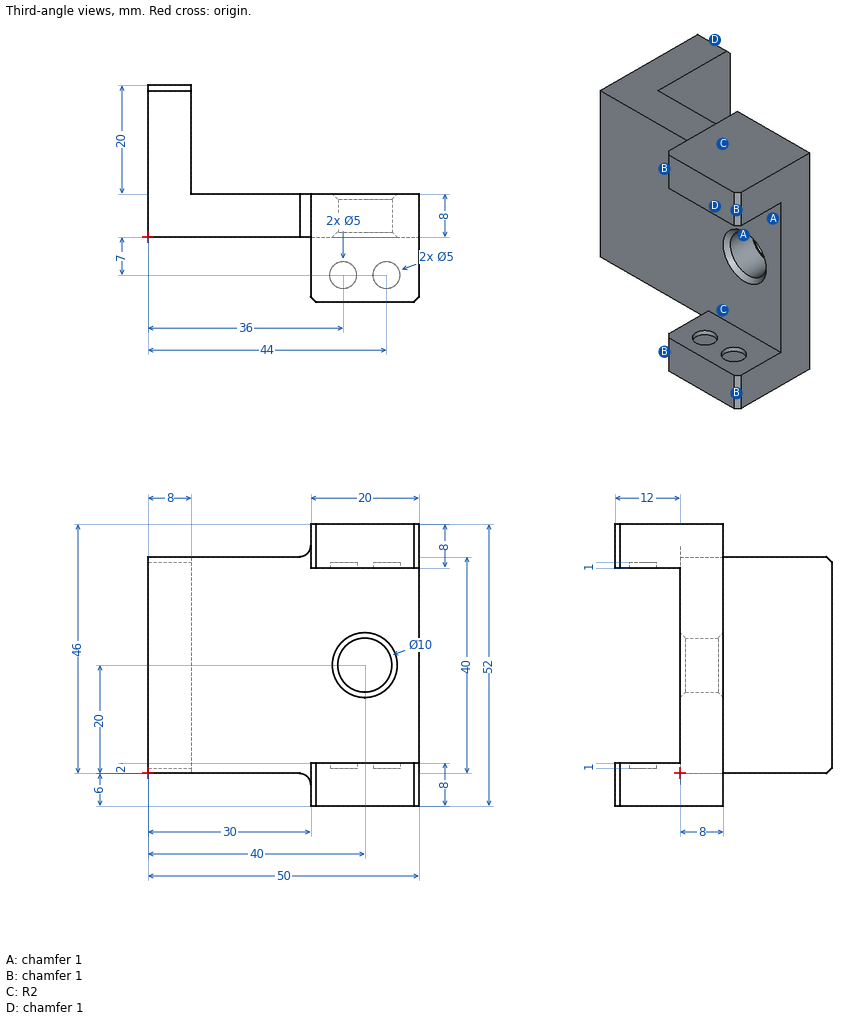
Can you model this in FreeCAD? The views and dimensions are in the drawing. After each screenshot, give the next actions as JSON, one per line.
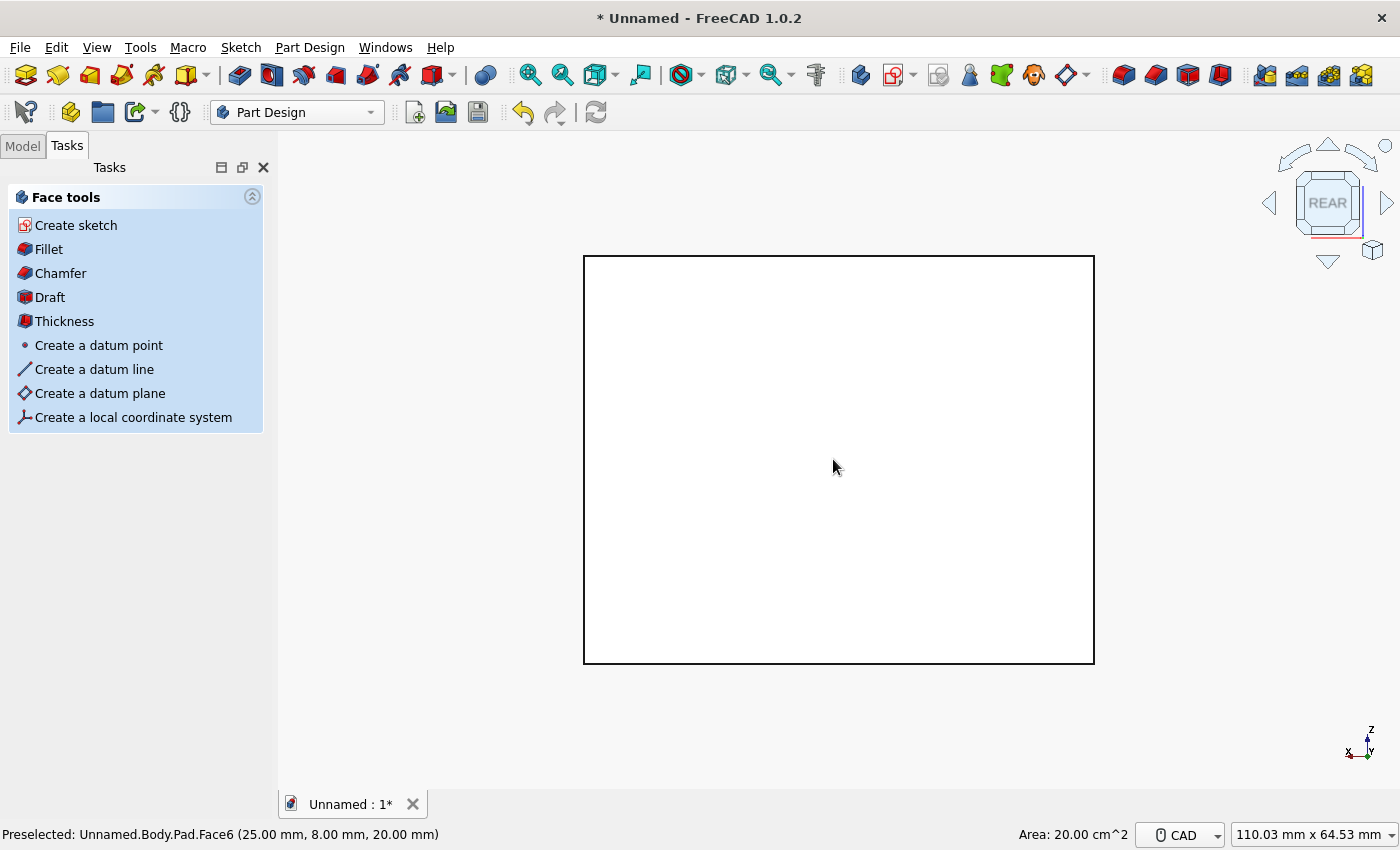
{"action": "left_click", "coordinate": [894, 76]}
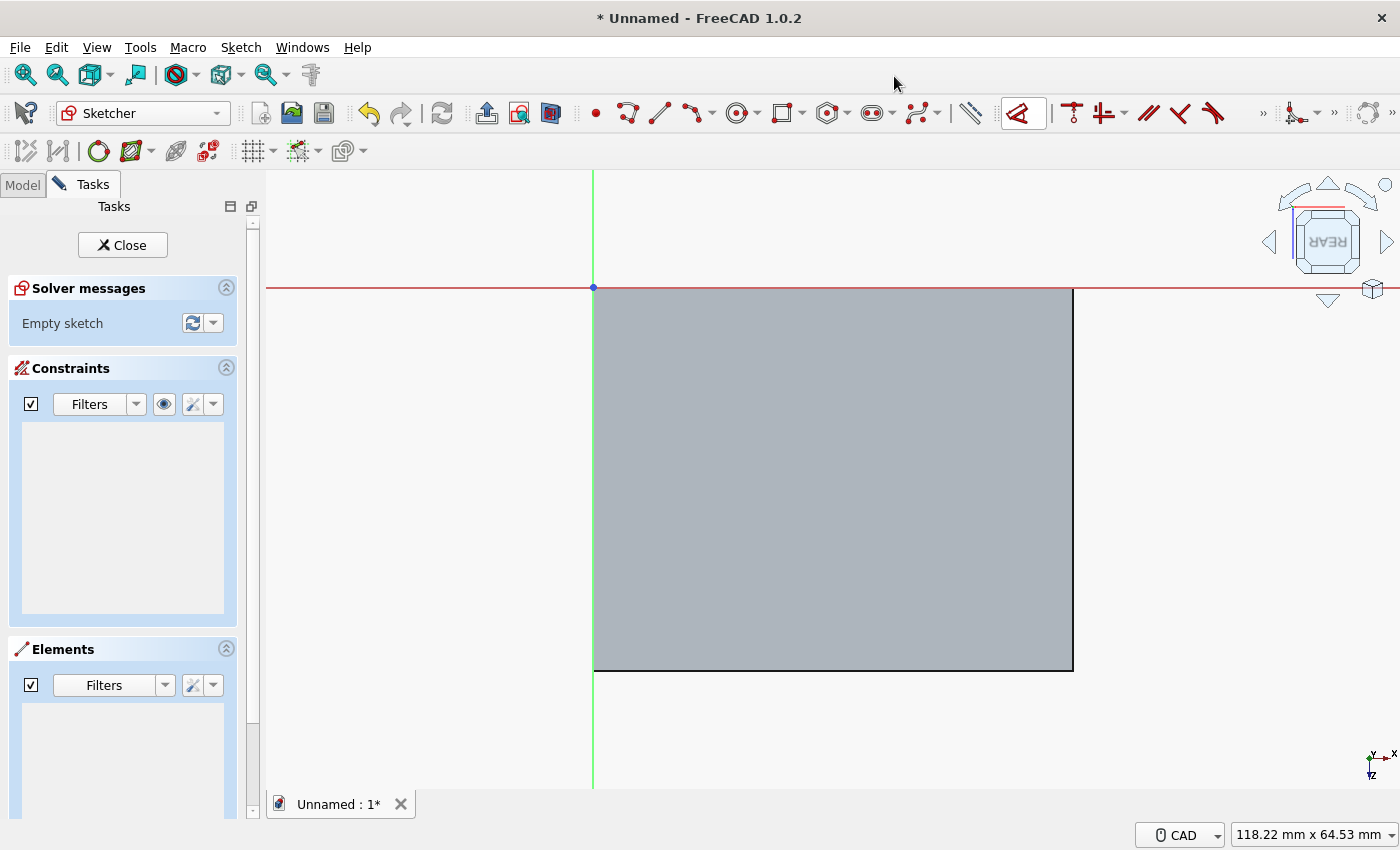
{"action": "key", "text": "g r"}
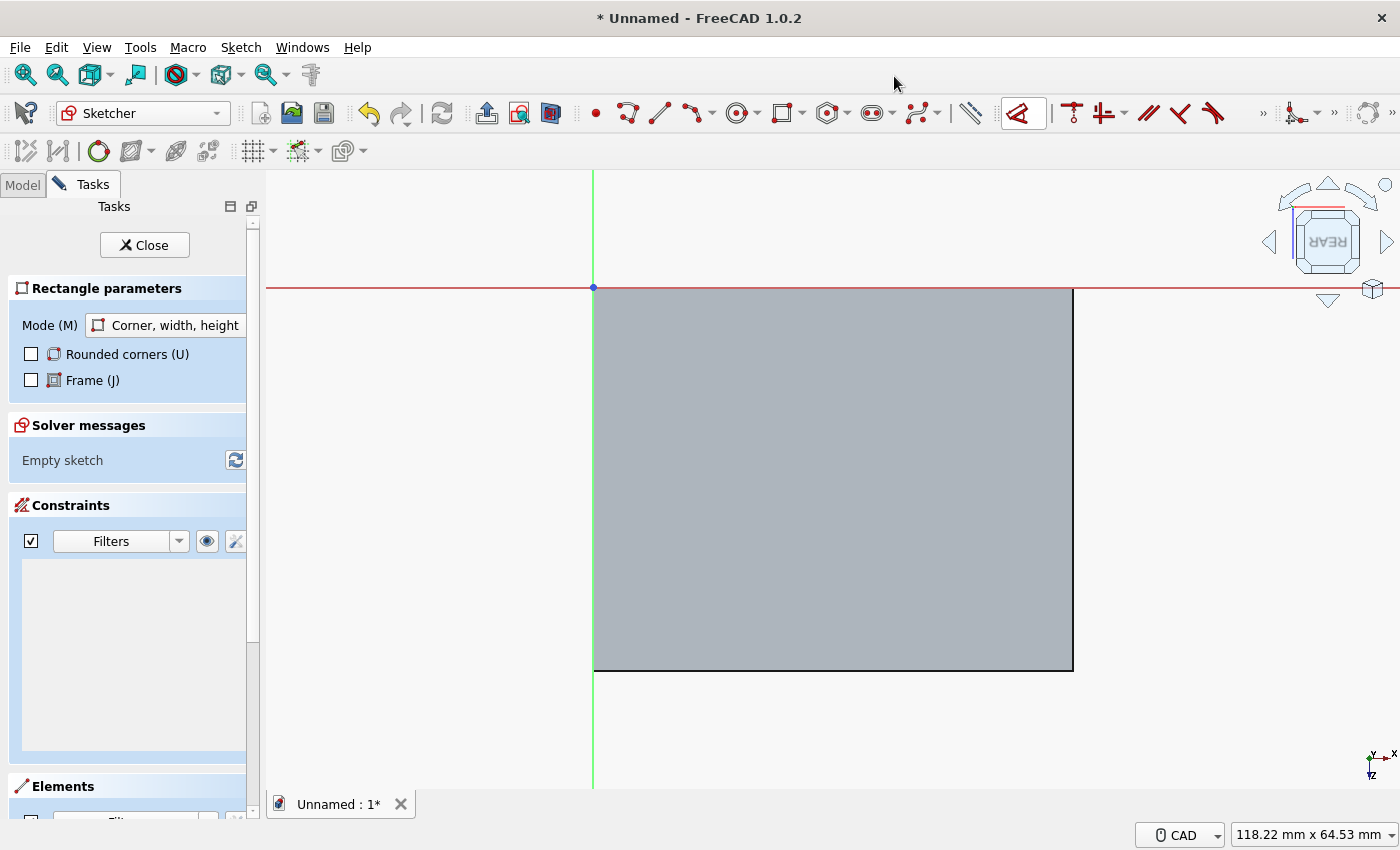
{"action": "left_click", "coordinate": [881, 230]}
{"action": "mouse_move", "coordinate": [1073, 729]}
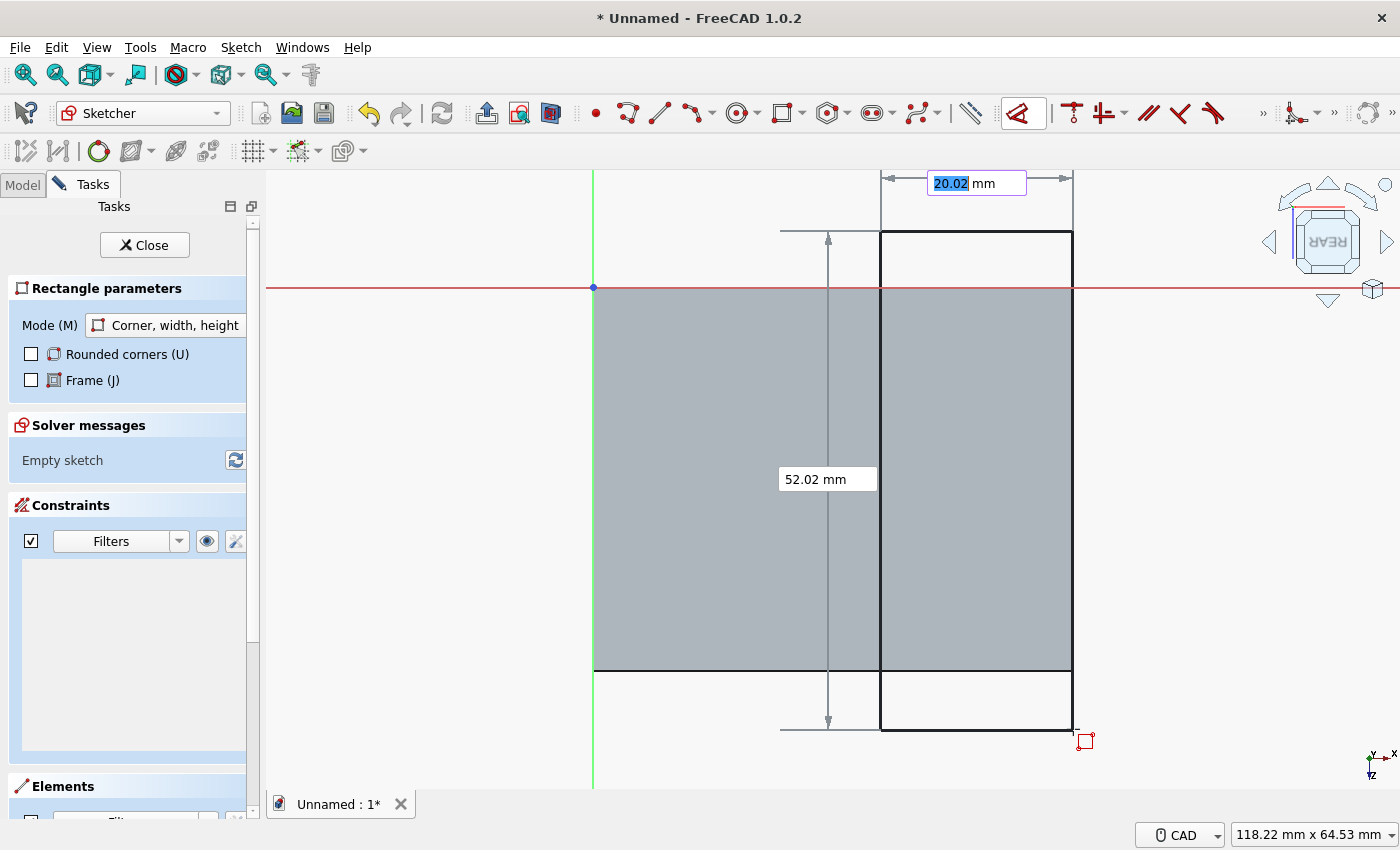
{"action": "type", "text": "20"}
{"action": "key", "text": "Tab"}
{"action": "type", "text": "52"}
{"action": "key", "text": "Return"}
{"action": "key", "text": "Escape"}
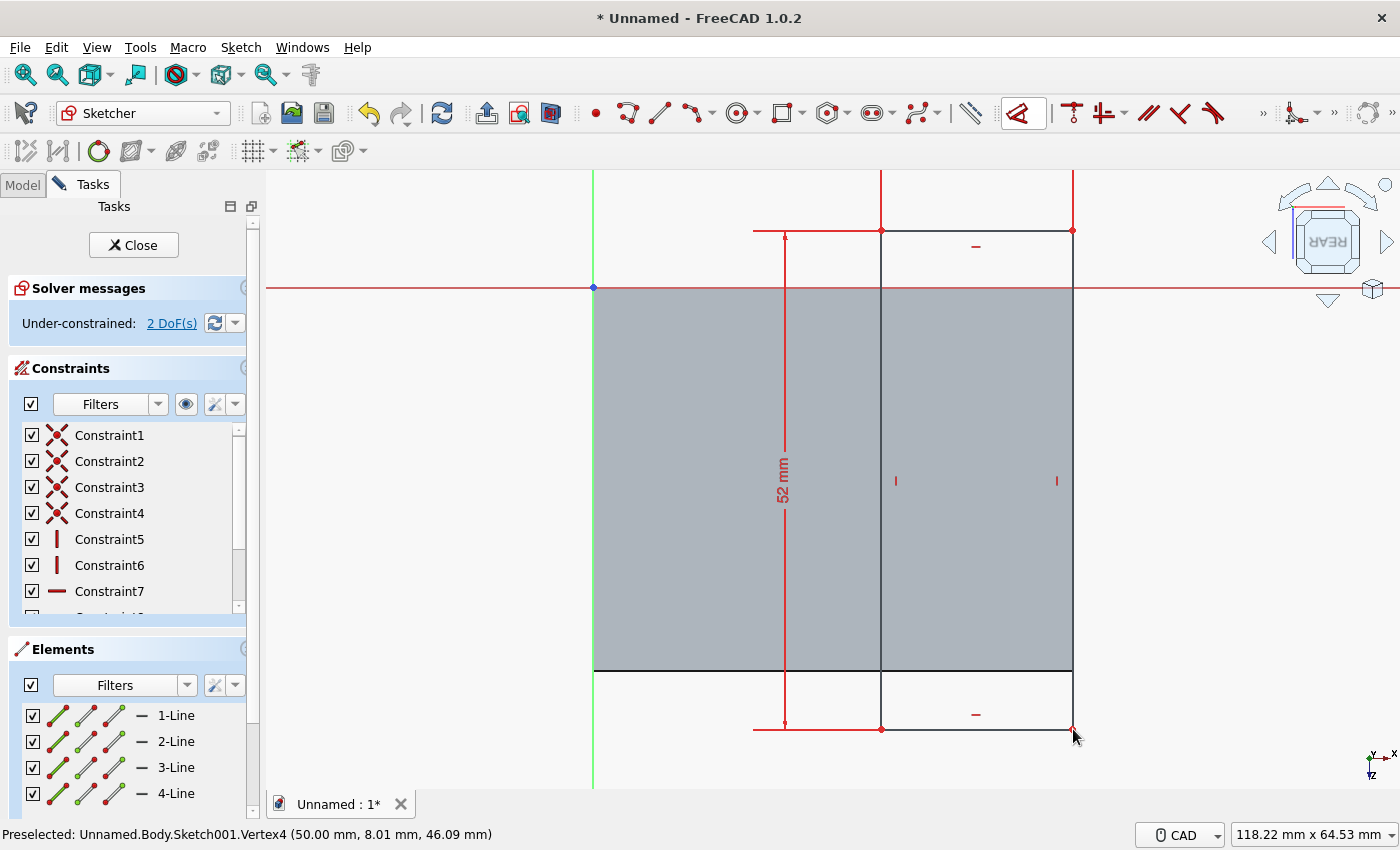
{"action": "left_click", "coordinate": [1018, 114]}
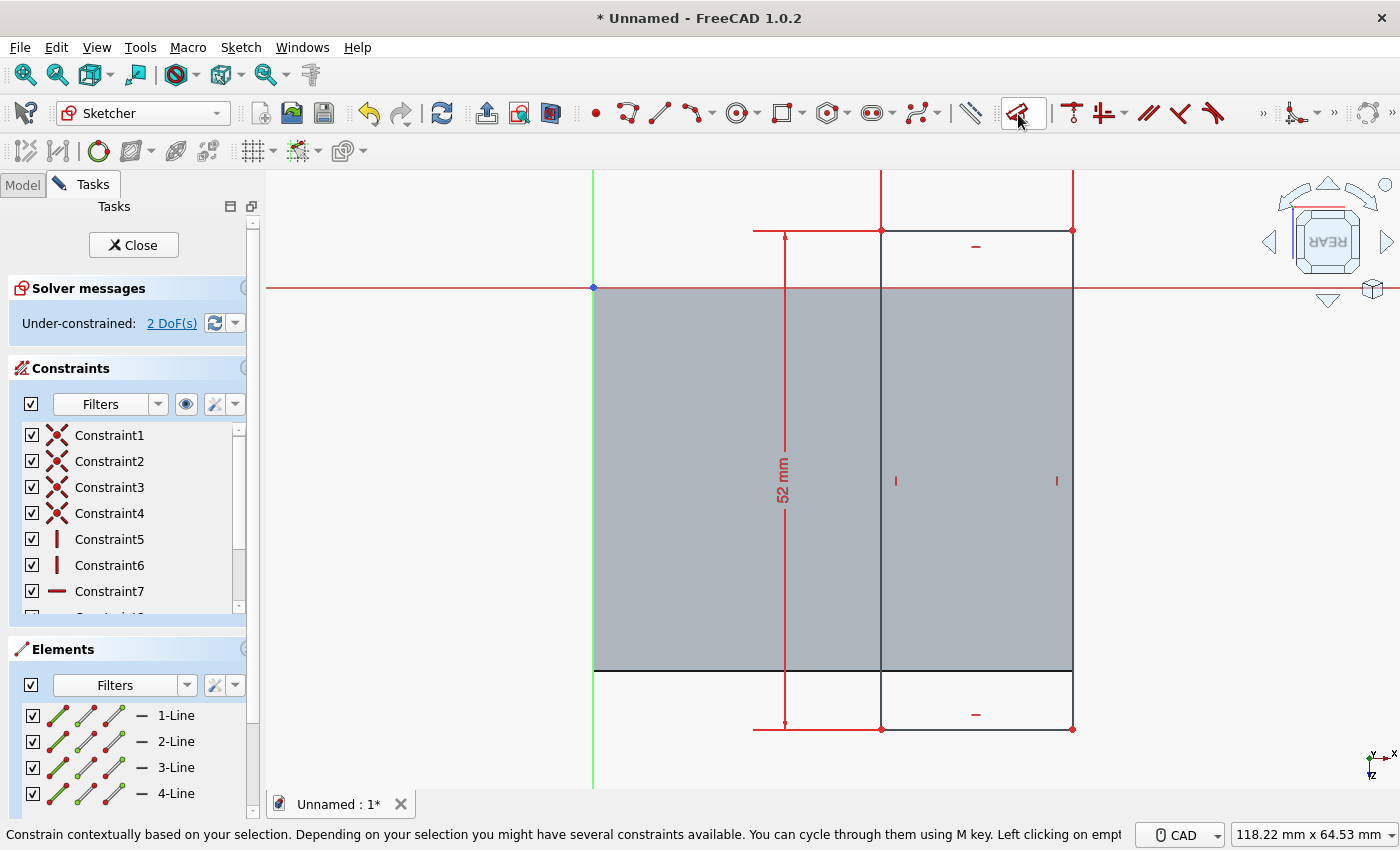
{"action": "left_click", "coordinate": [881, 231]}
{"action": "left_click", "coordinate": [559, 259]}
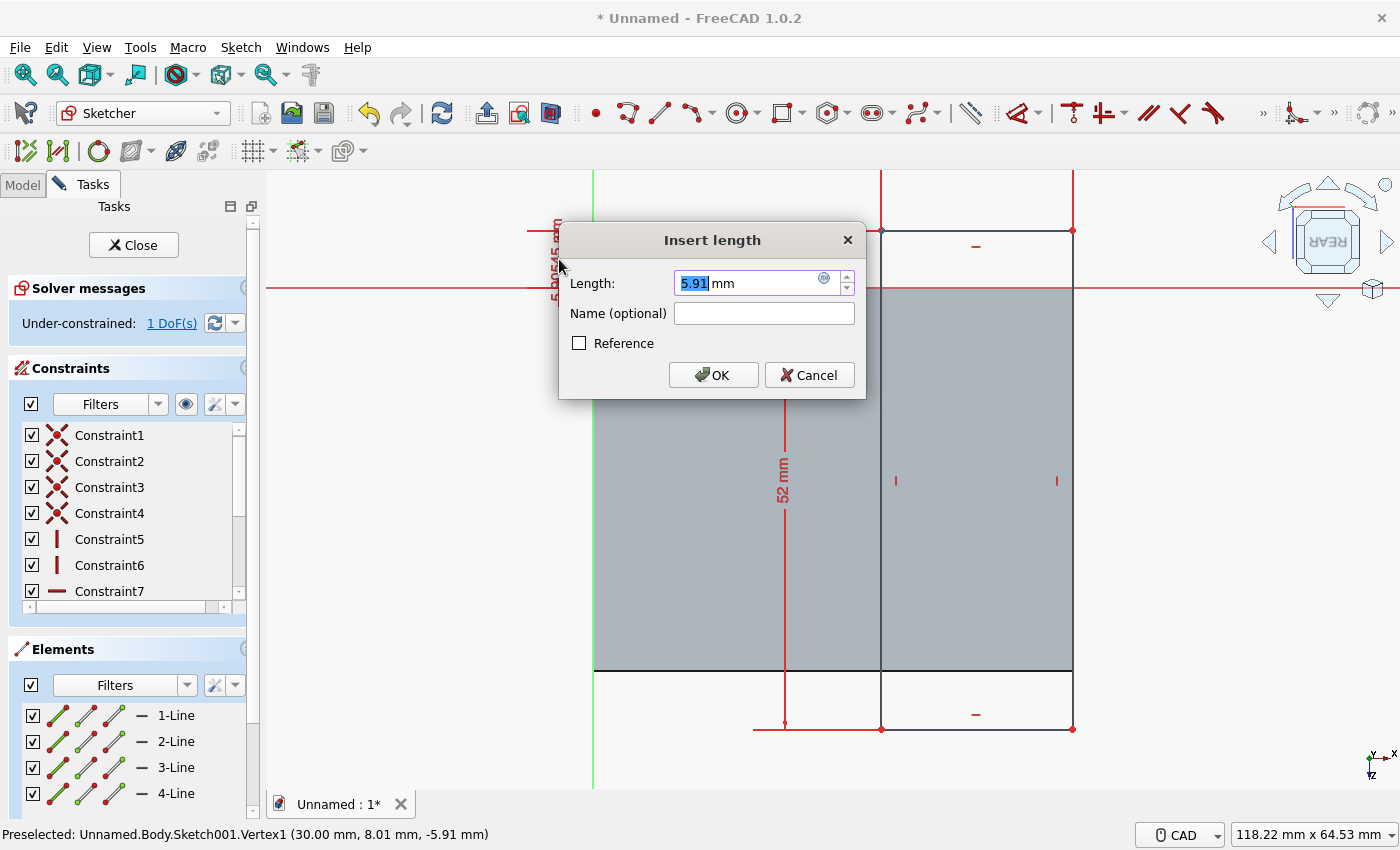
{"action": "type", "text": "6"}
{"action": "key", "text": "Return"}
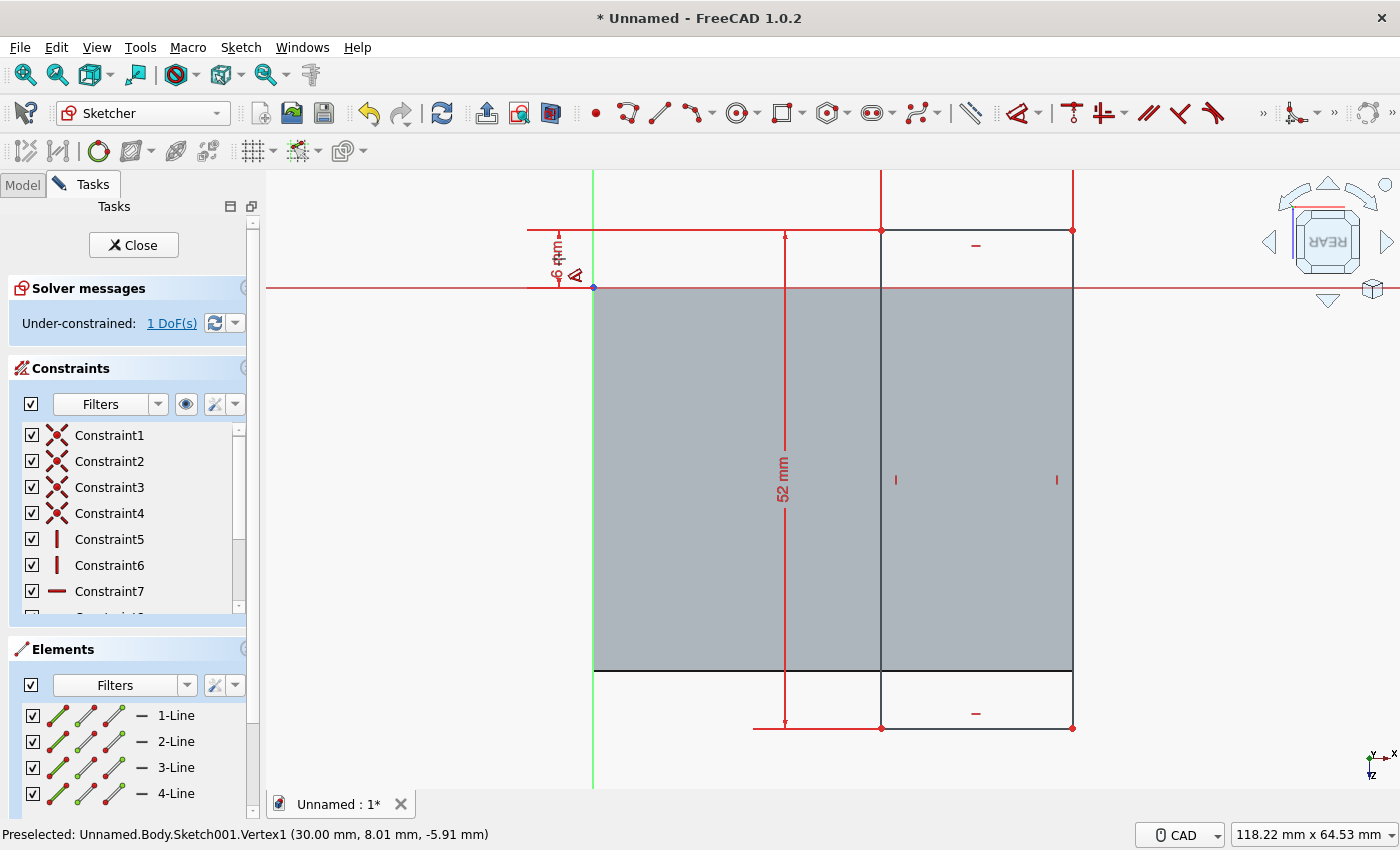
{"action": "left_click", "coordinate": [881, 230]}
{"action": "left_click", "coordinate": [737, 322]}